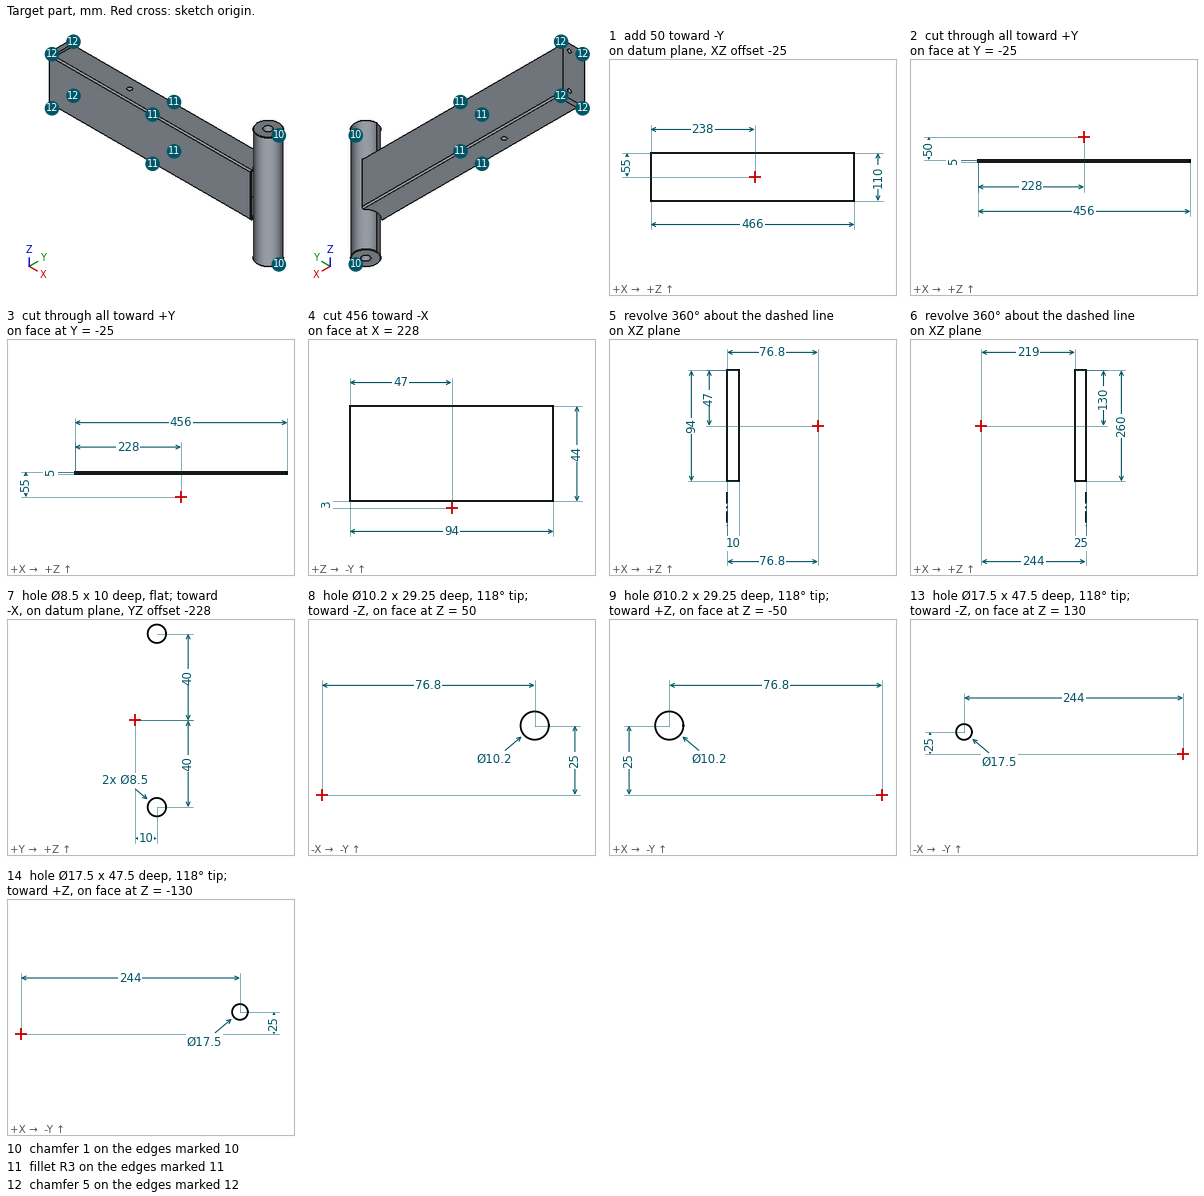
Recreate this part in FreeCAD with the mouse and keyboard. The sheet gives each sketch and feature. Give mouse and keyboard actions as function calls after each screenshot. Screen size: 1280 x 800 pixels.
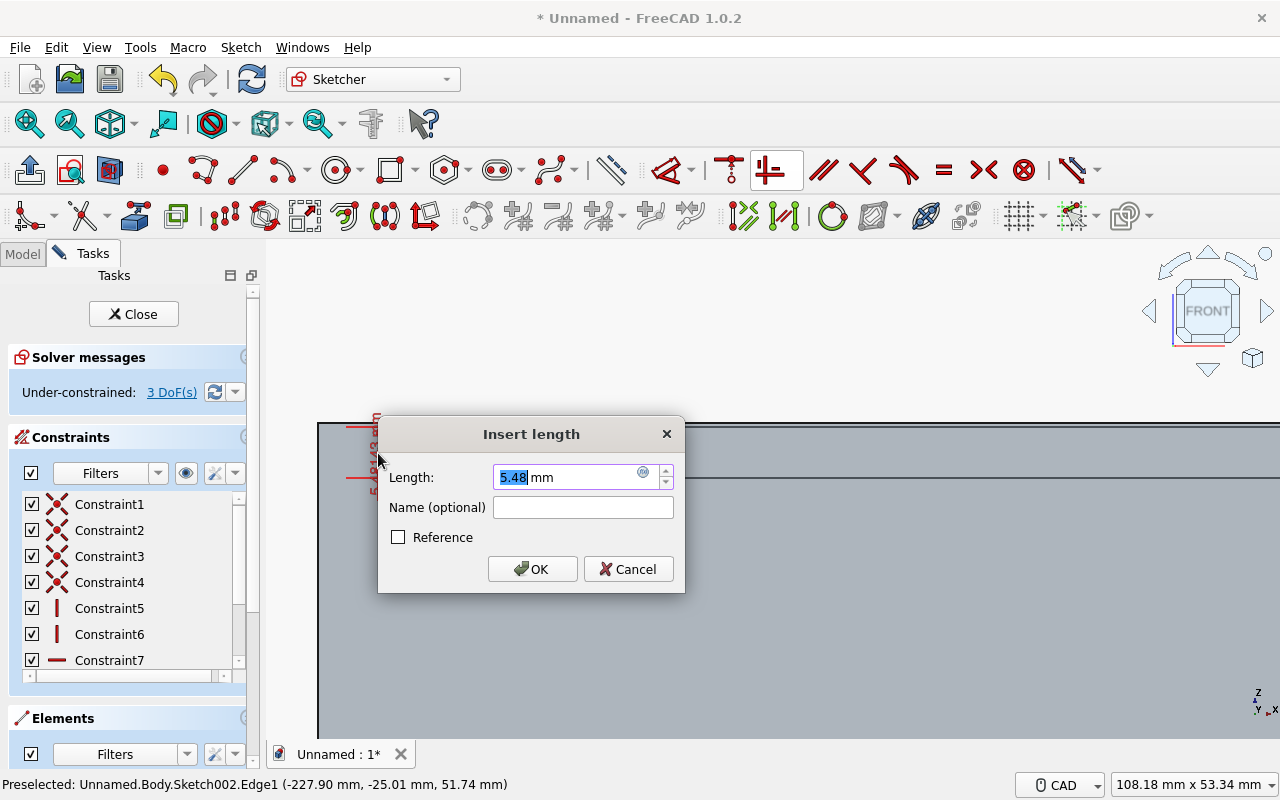
text(5)
key(Return)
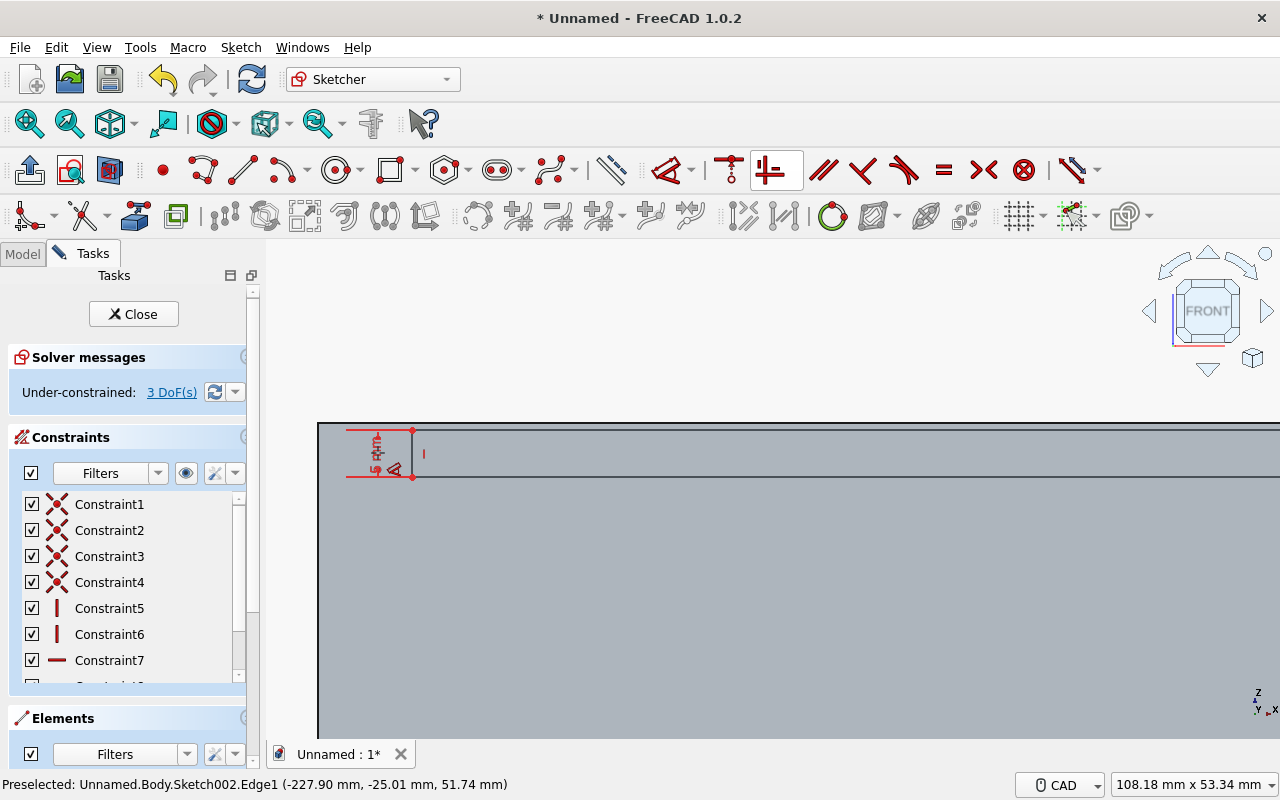
scroll(416, 459, down, 10)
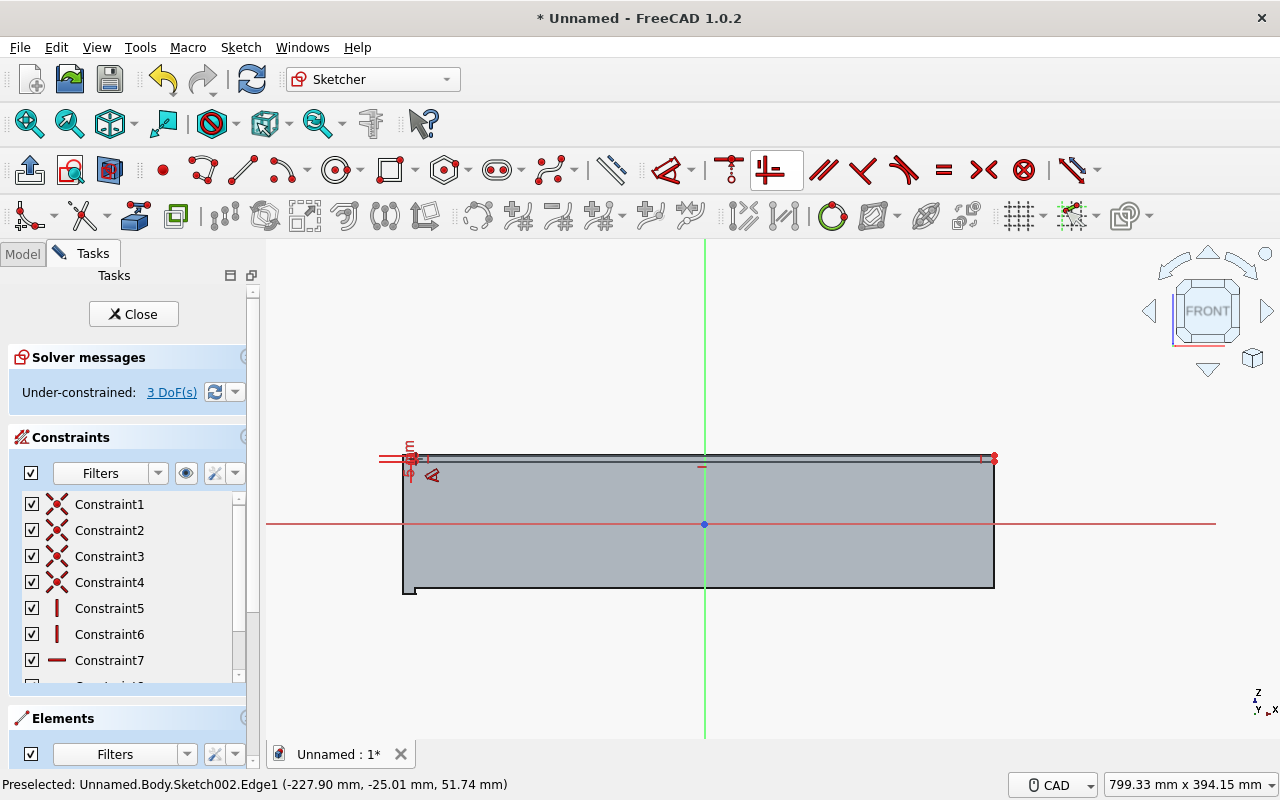
scroll(589, 462, up, 4)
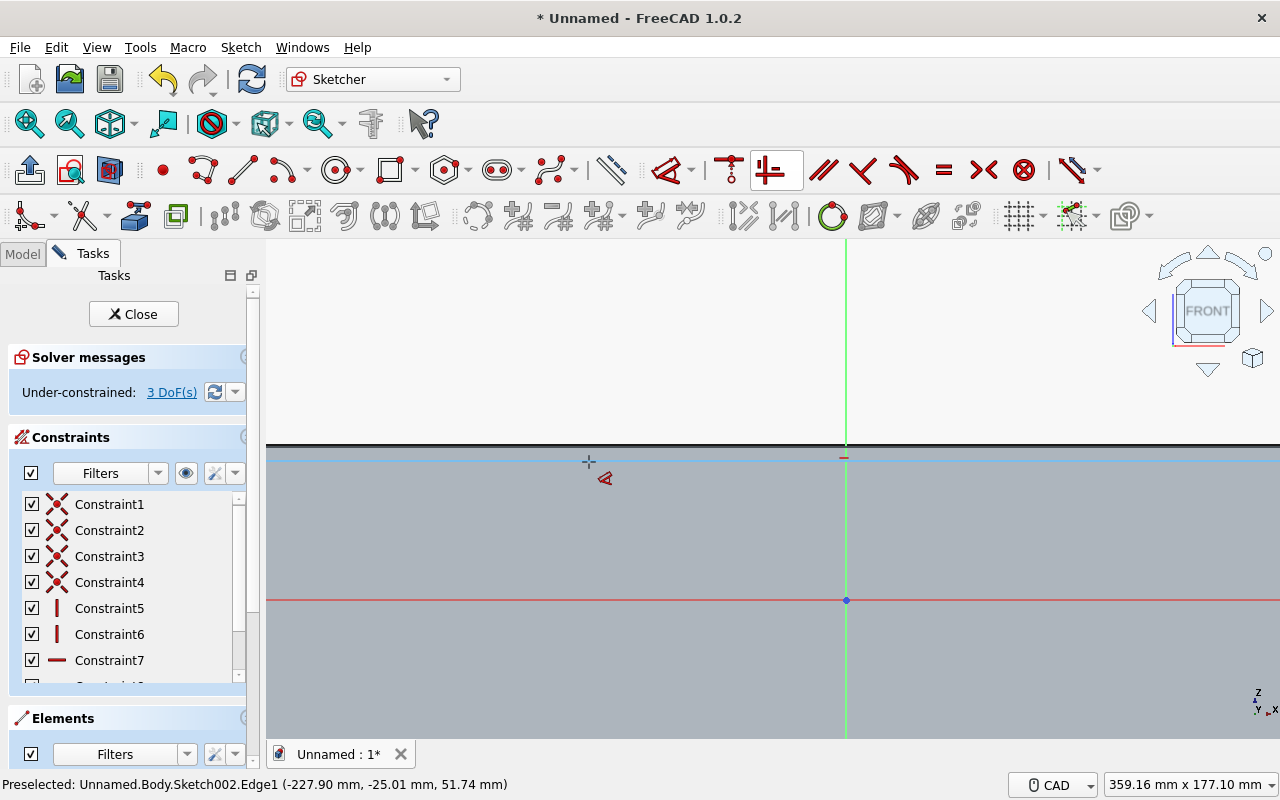
click(589, 461)
click(704, 427)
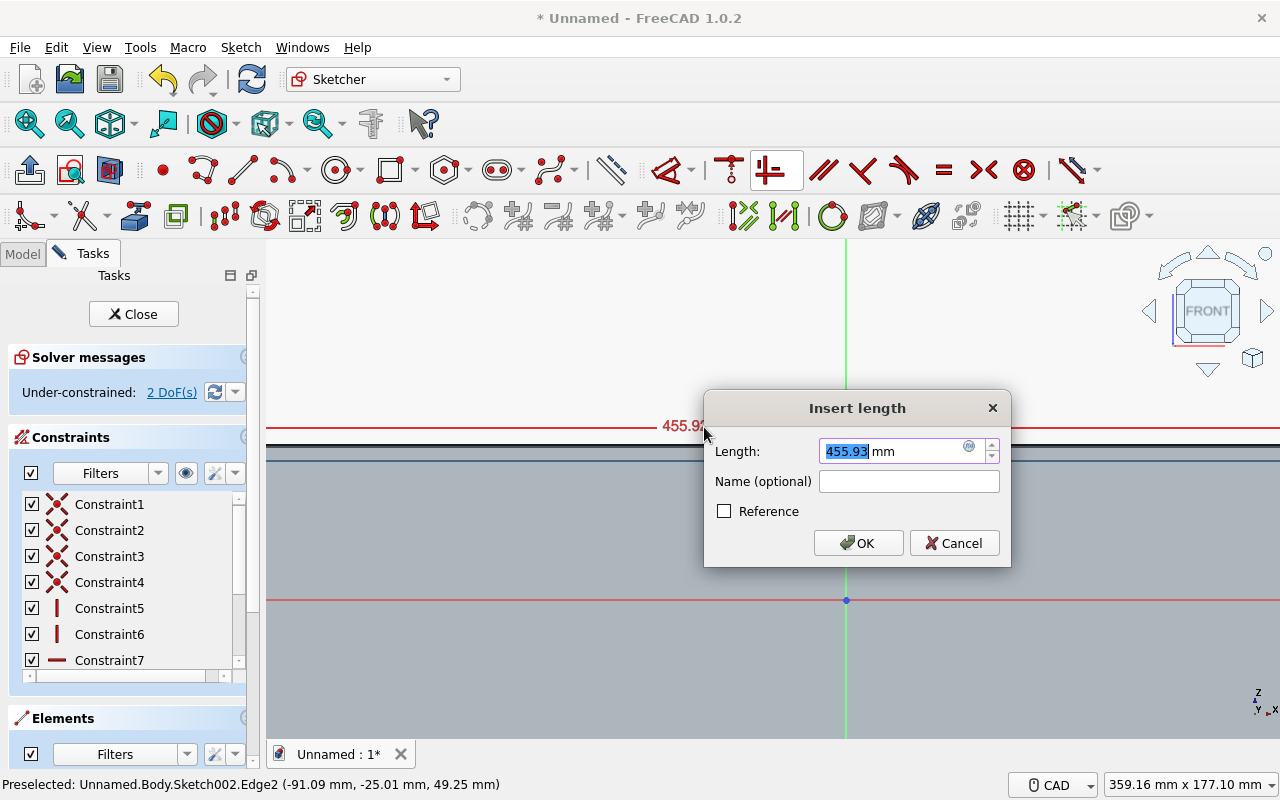
text(456)
key(Return)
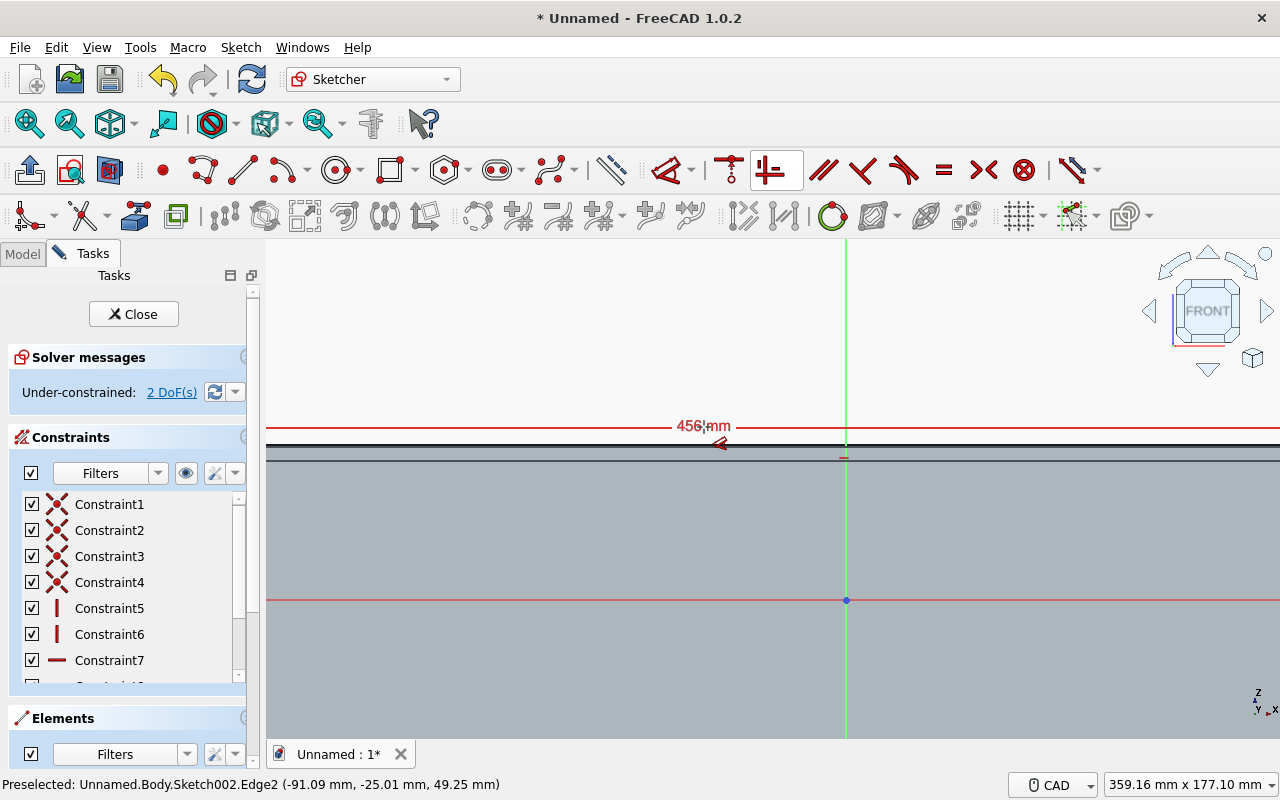
scroll(589, 462, down, 4)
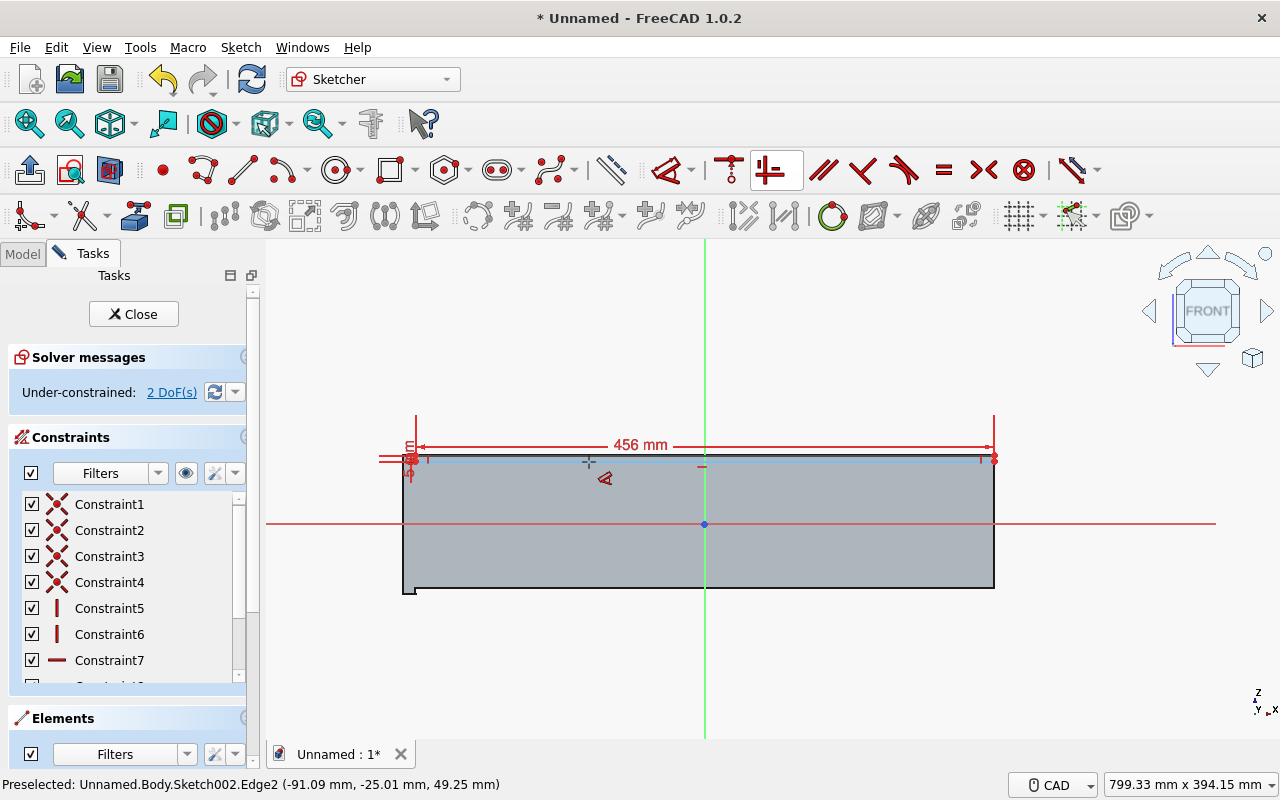
scroll(416, 456, up, 4)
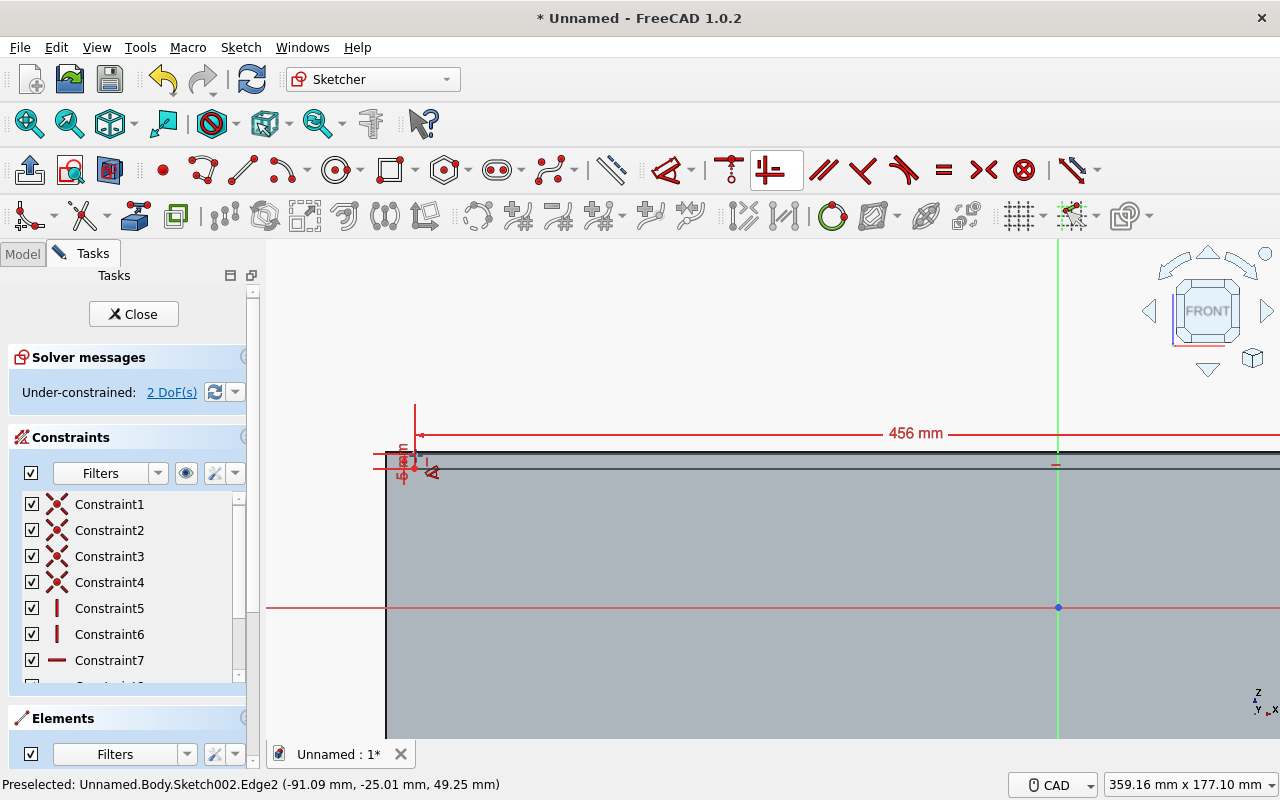
click(415, 454)
click(381, 531)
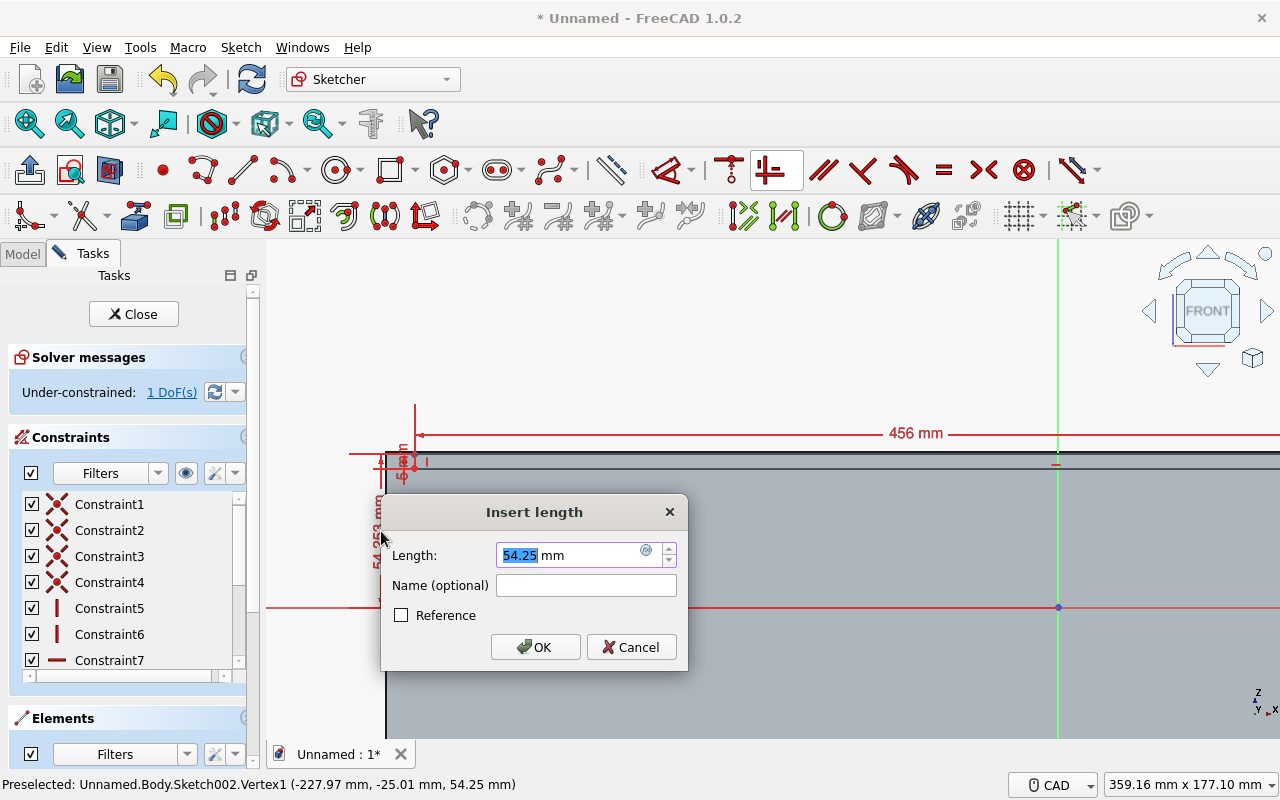
text(55)
key(Return)